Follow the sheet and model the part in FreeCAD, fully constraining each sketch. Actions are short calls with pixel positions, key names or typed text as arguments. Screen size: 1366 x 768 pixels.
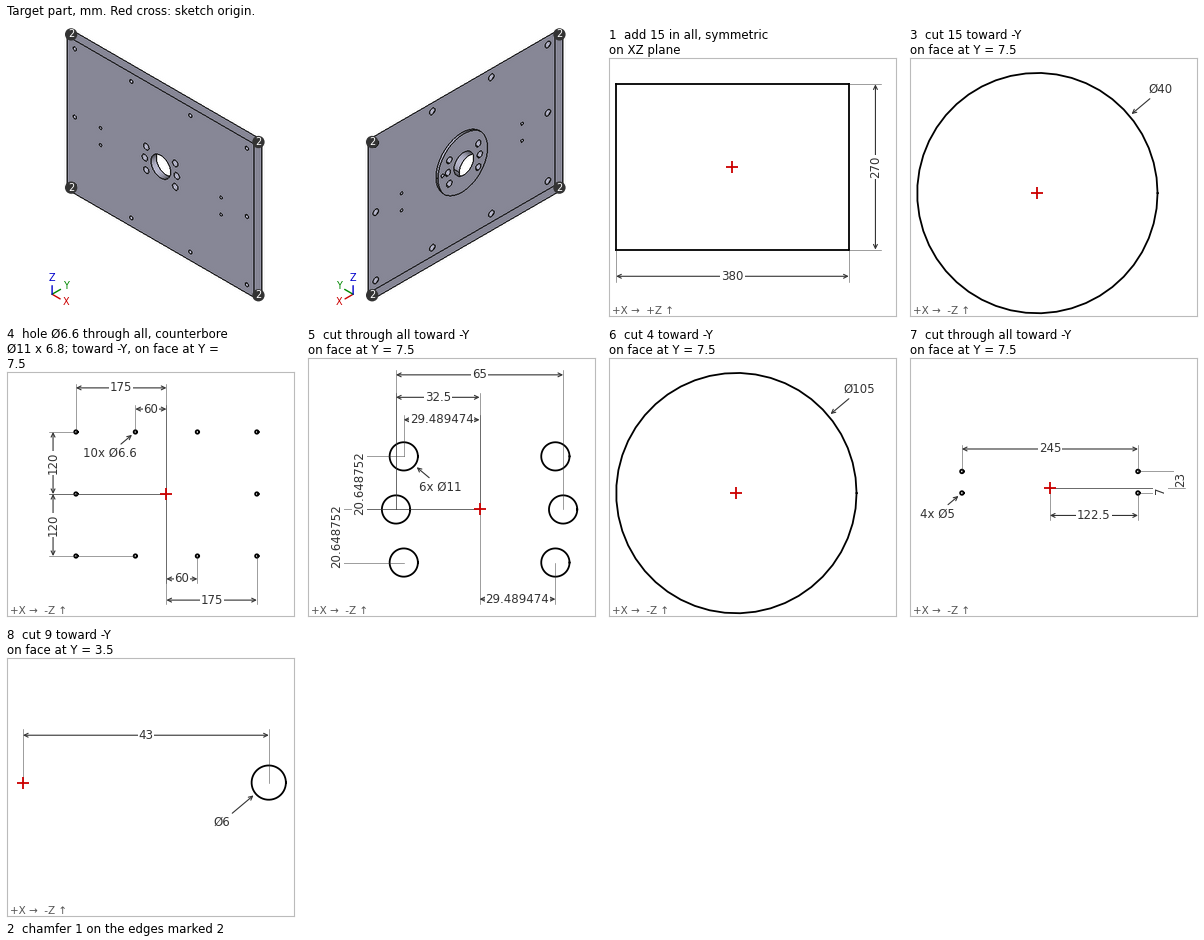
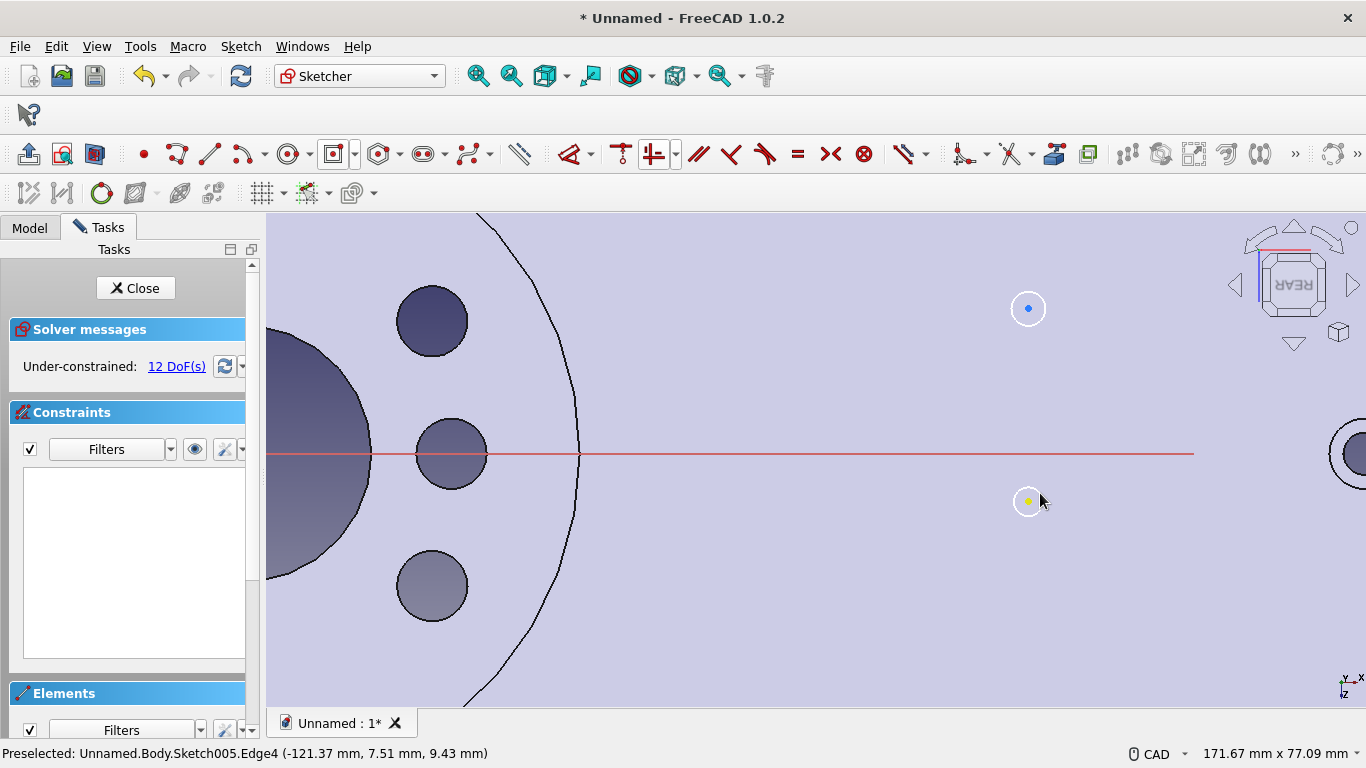
click(1038, 492)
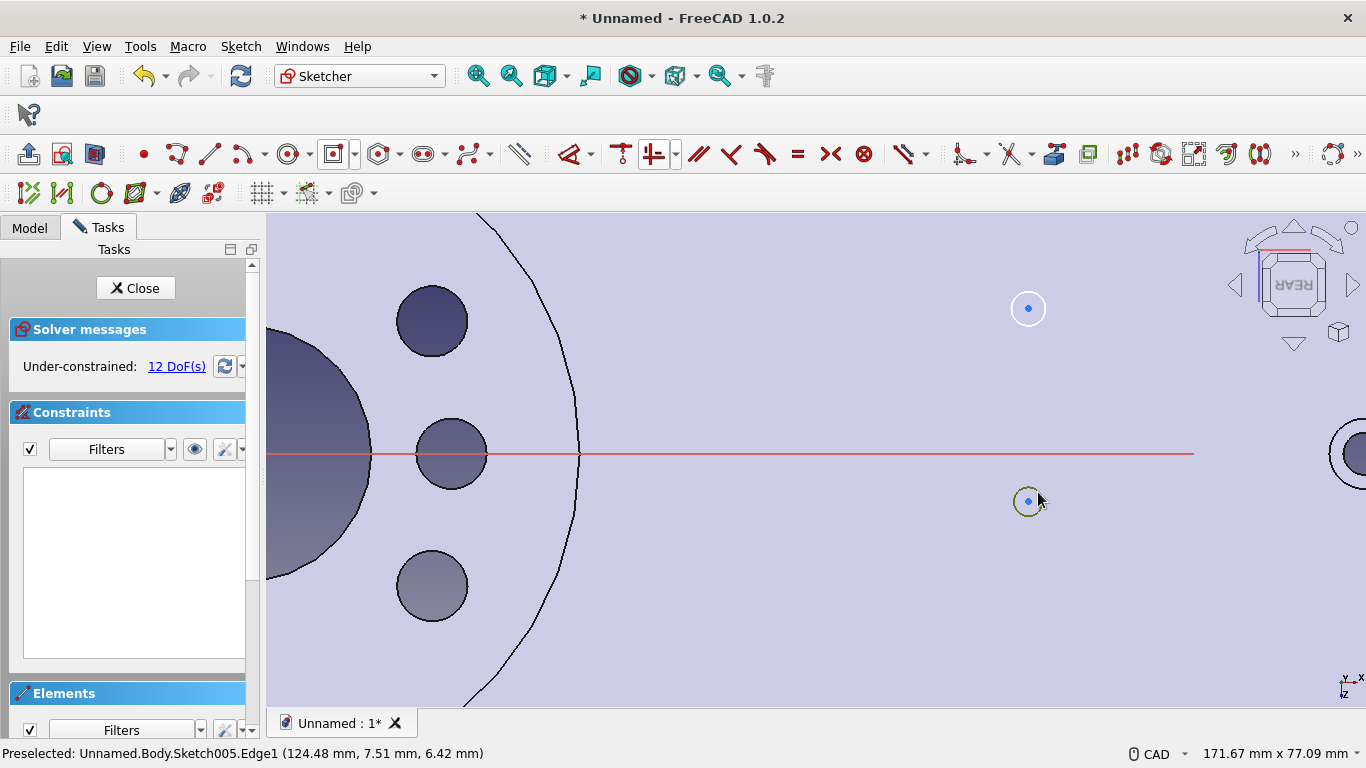
click(1040, 297)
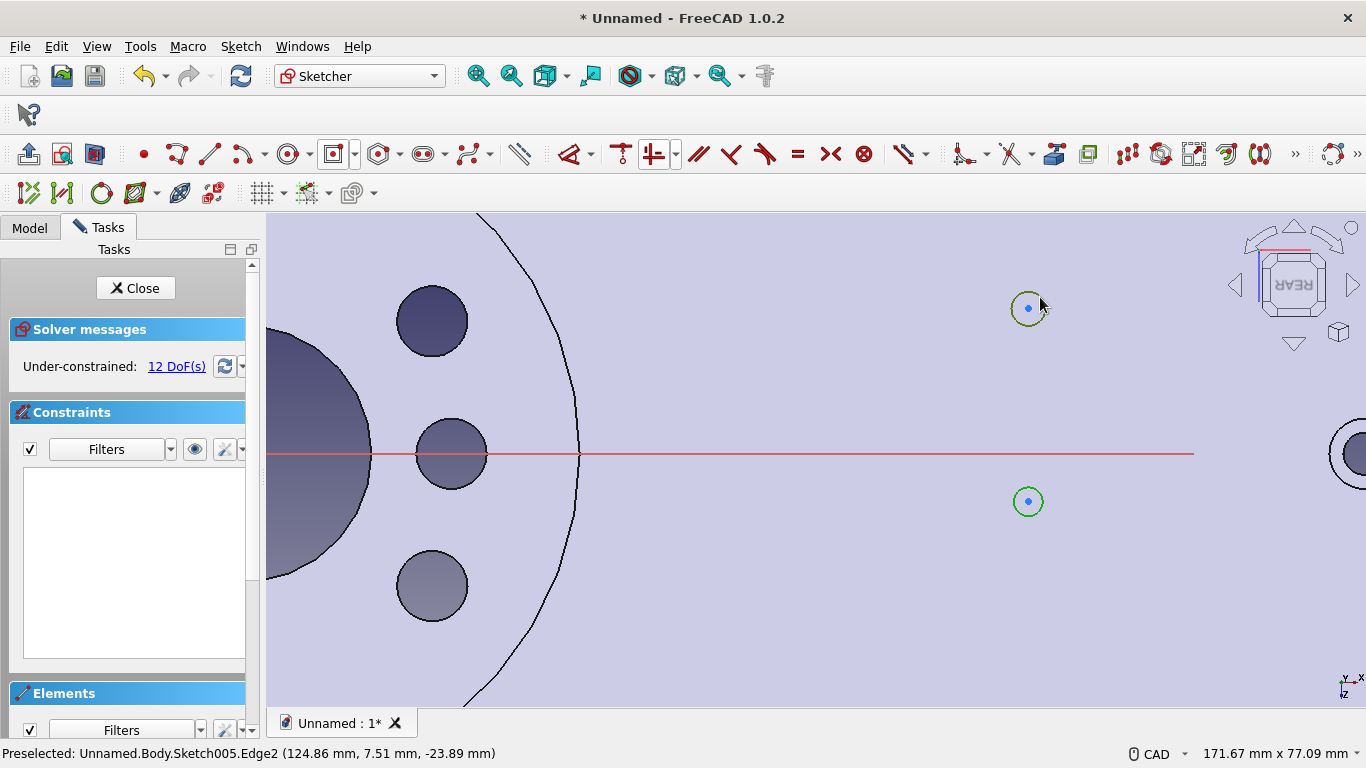
scroll(1041, 493, down, 5)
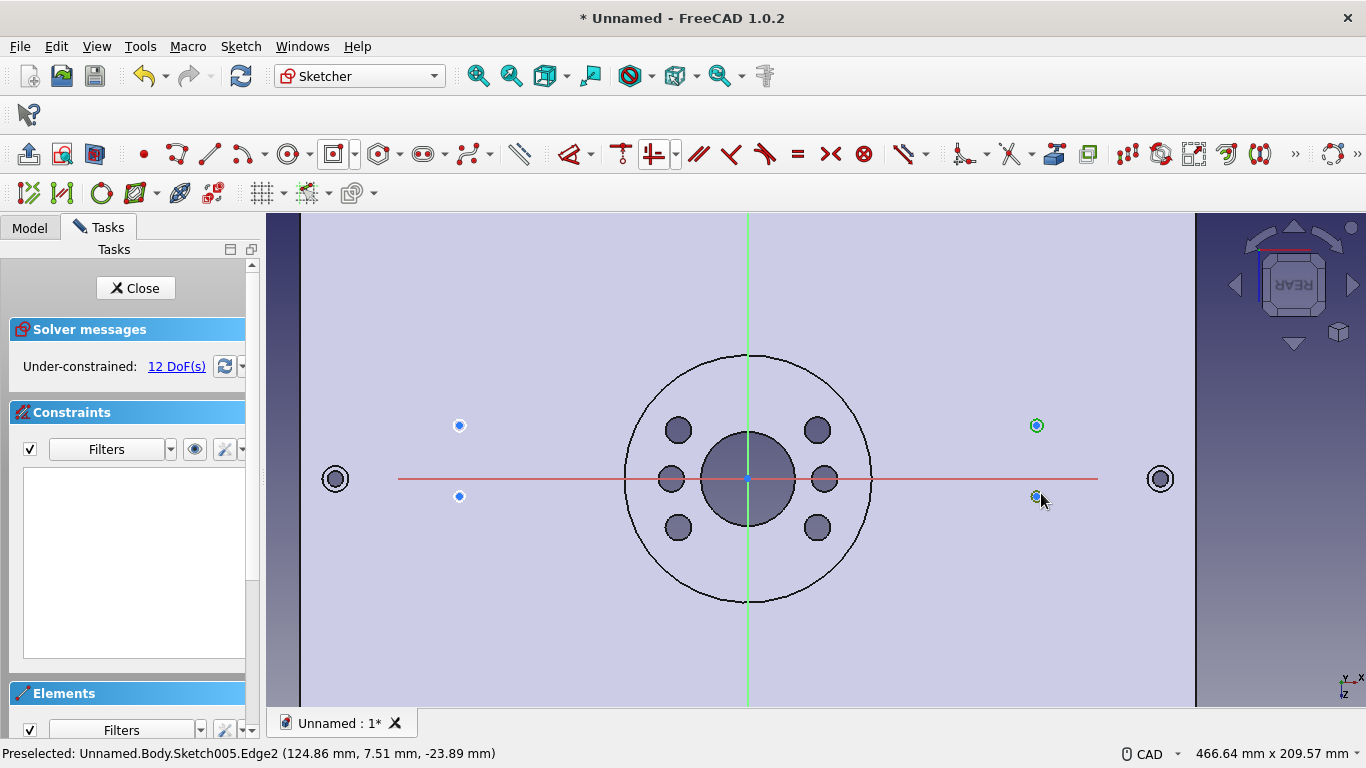
scroll(464, 421, up, 5)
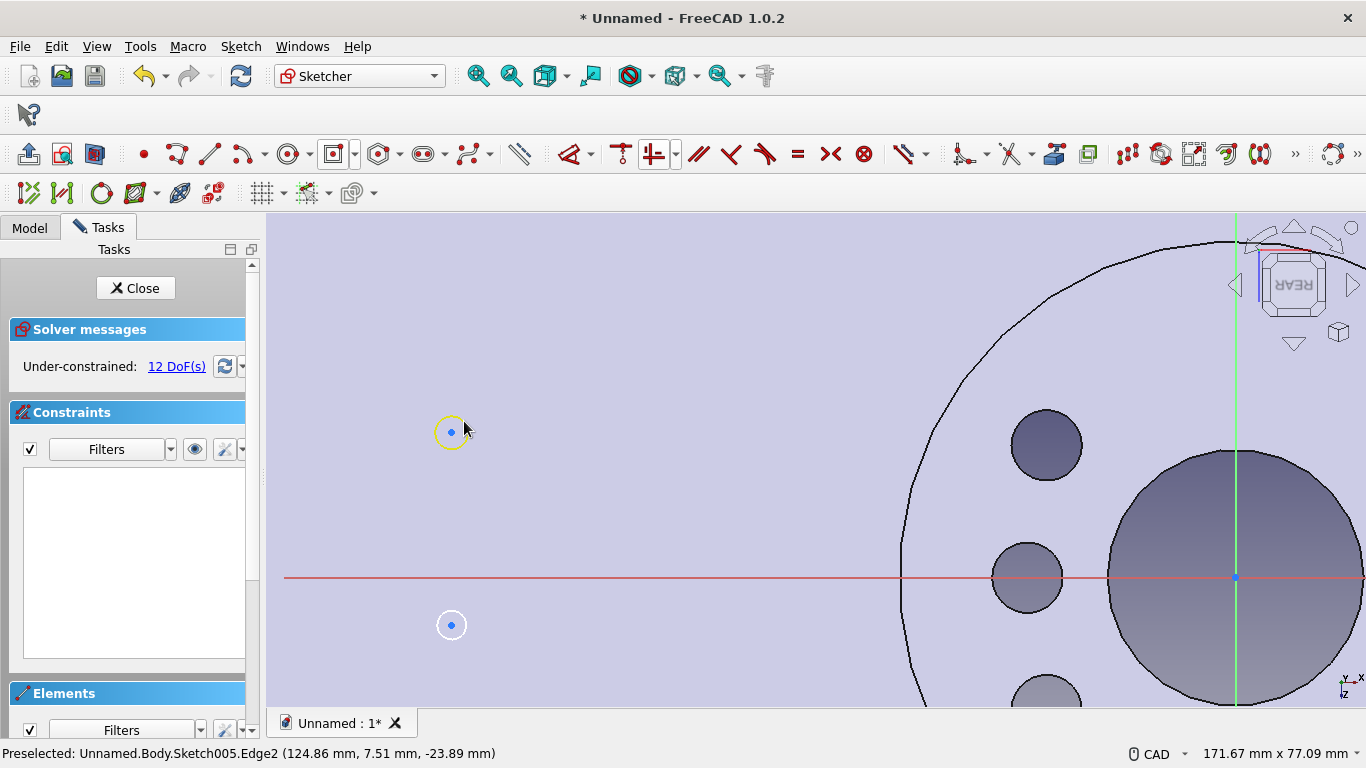
click(463, 421)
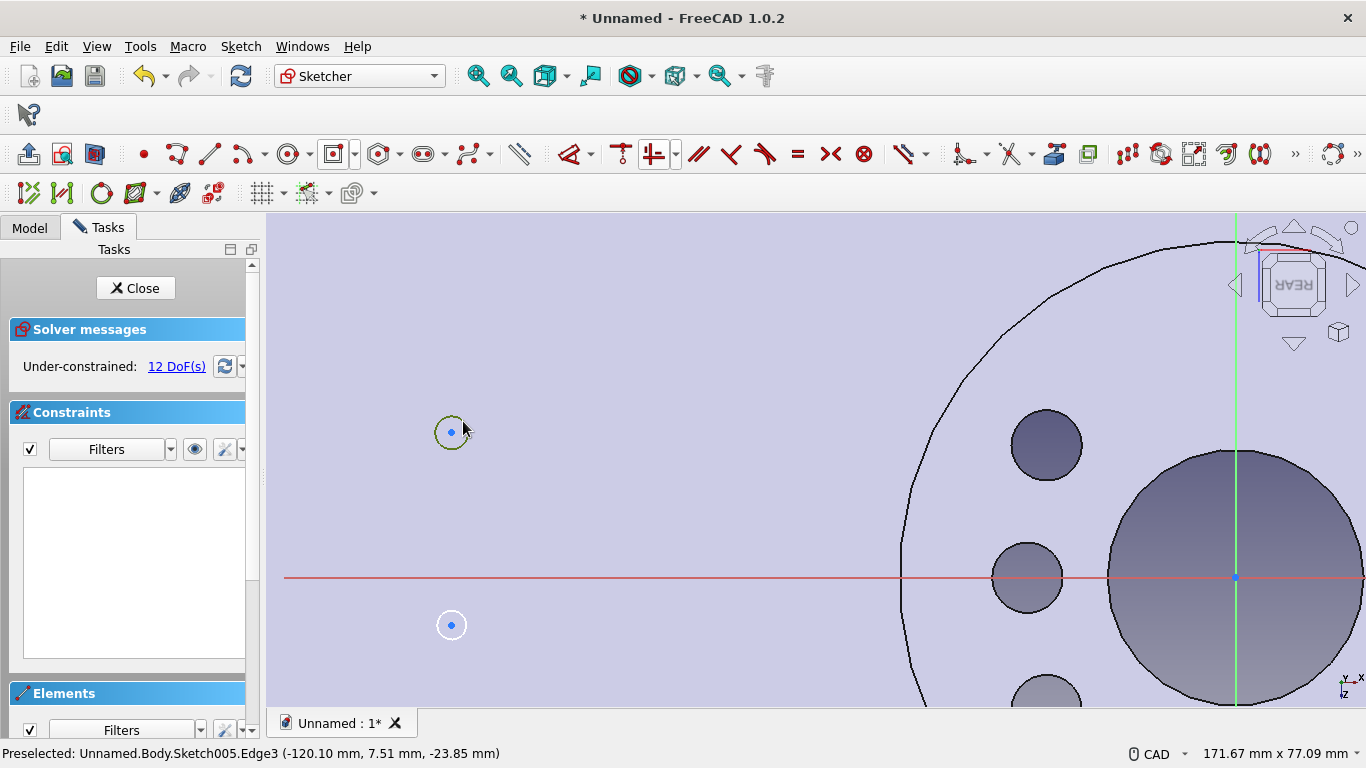
click(462, 615)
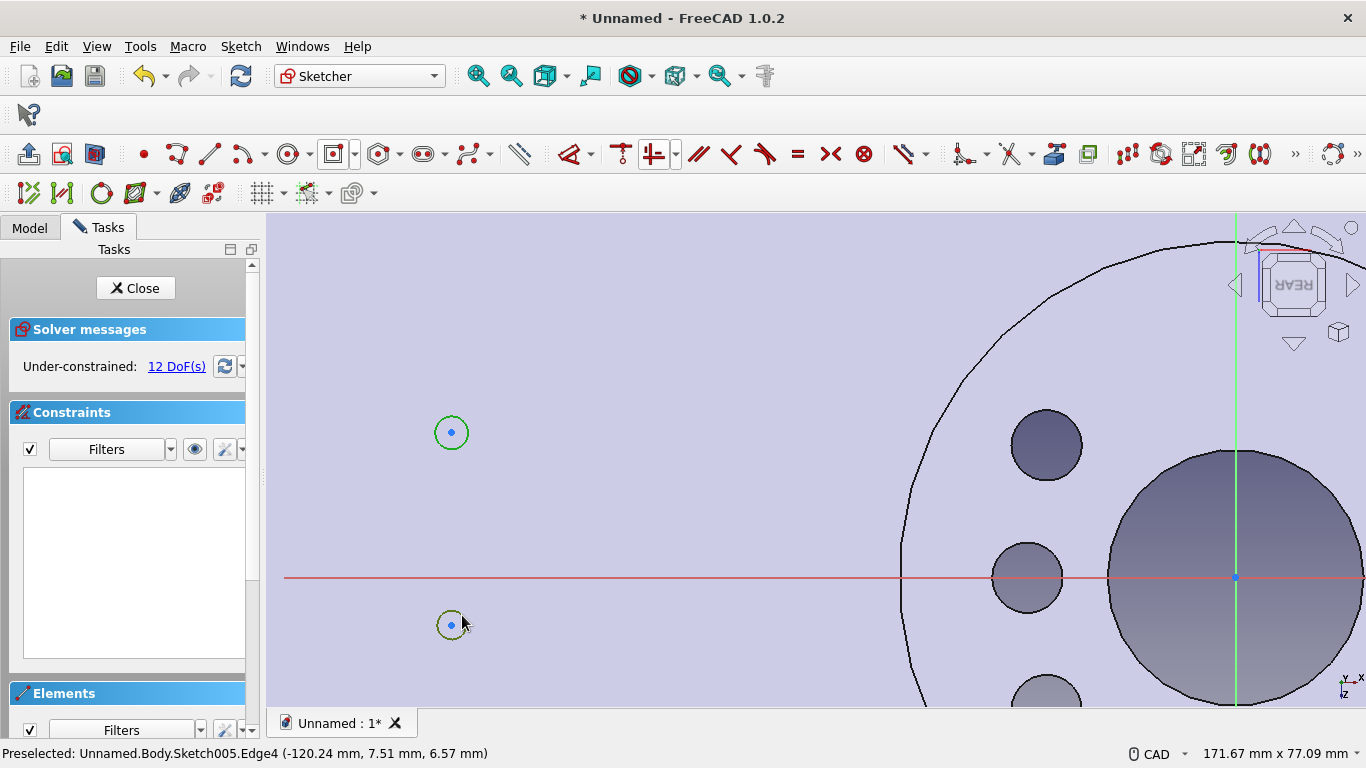
click(798, 154)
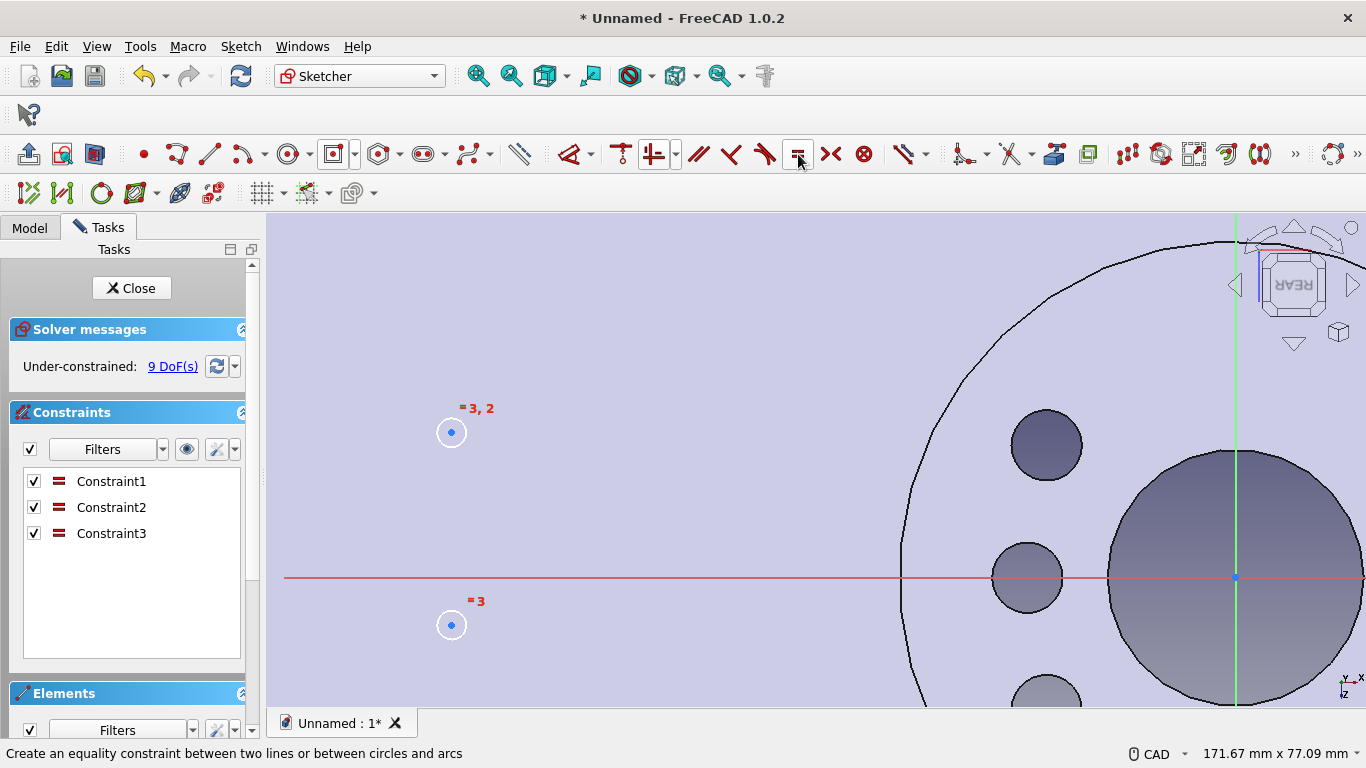
scroll(463, 421, down, 5)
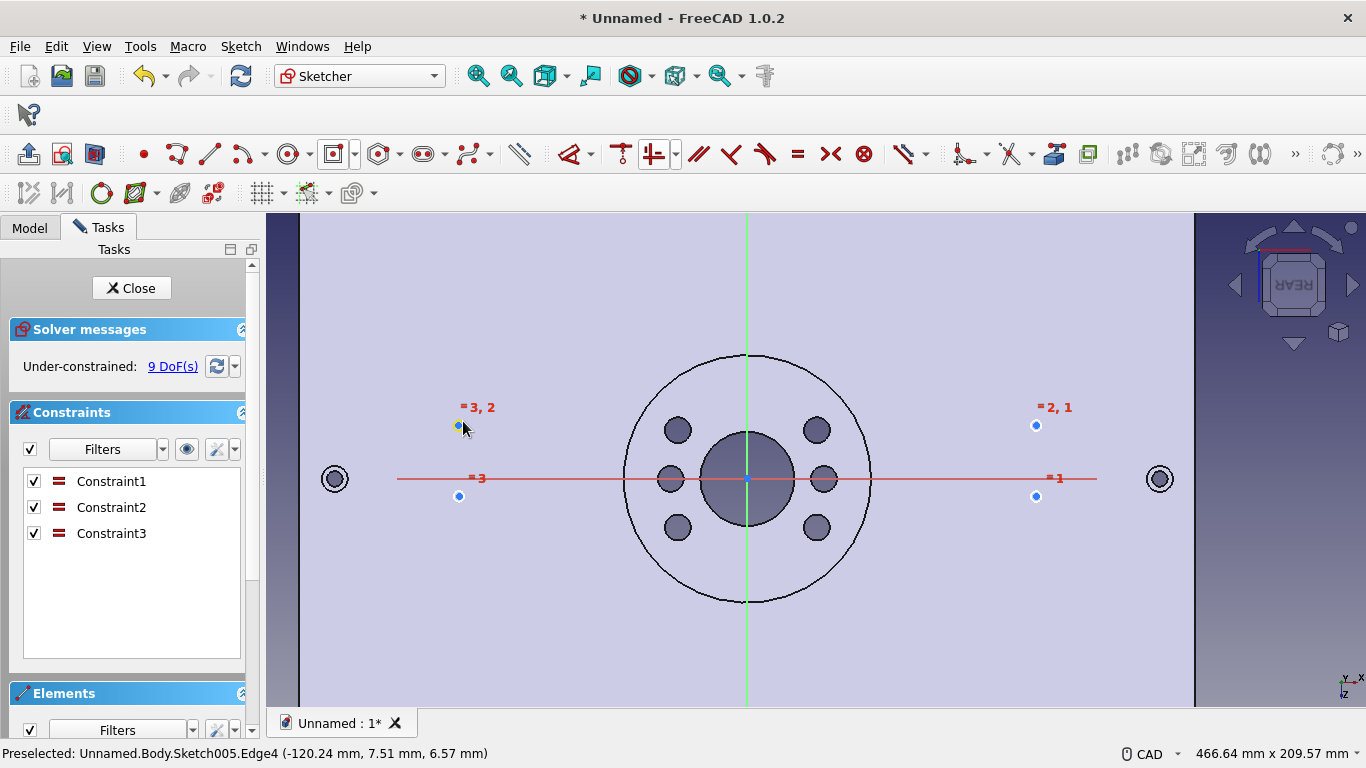
click(1036, 497)